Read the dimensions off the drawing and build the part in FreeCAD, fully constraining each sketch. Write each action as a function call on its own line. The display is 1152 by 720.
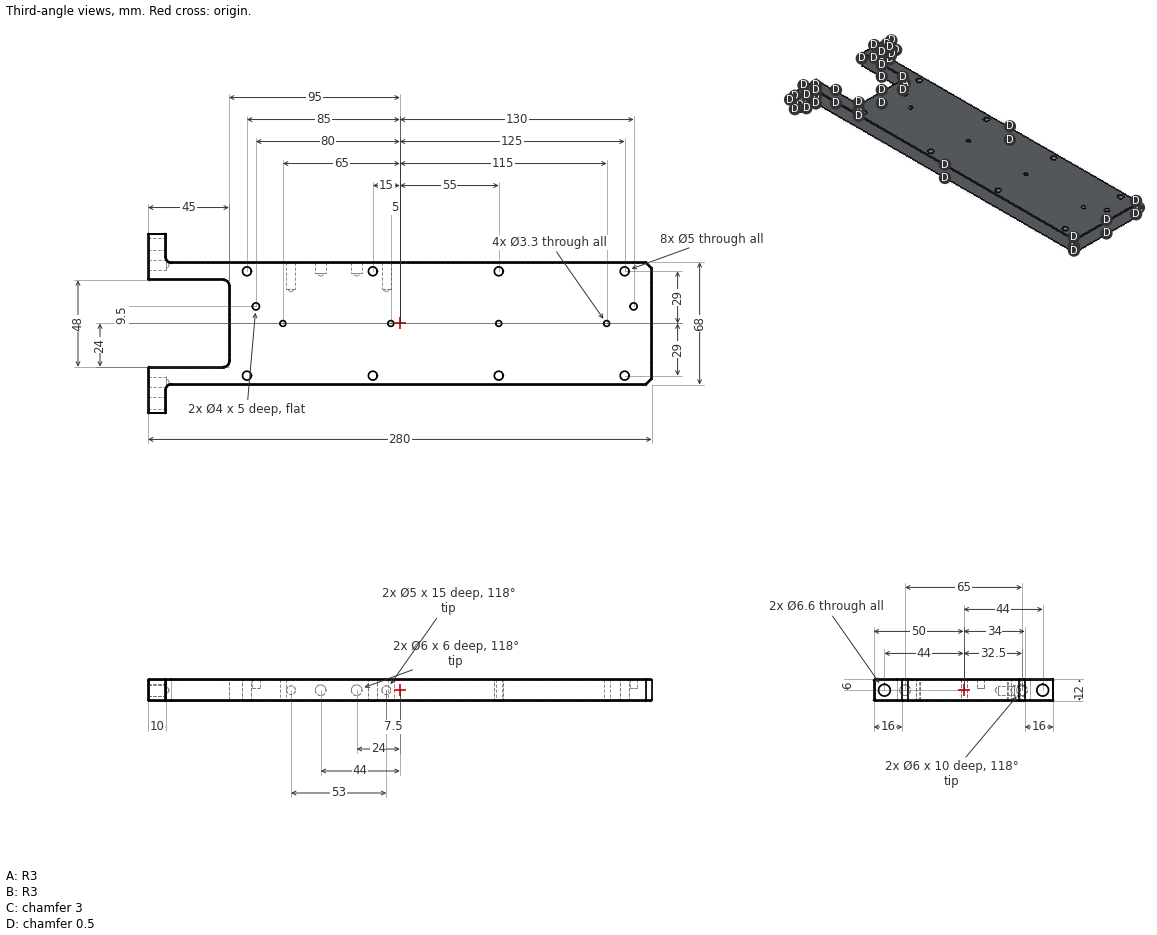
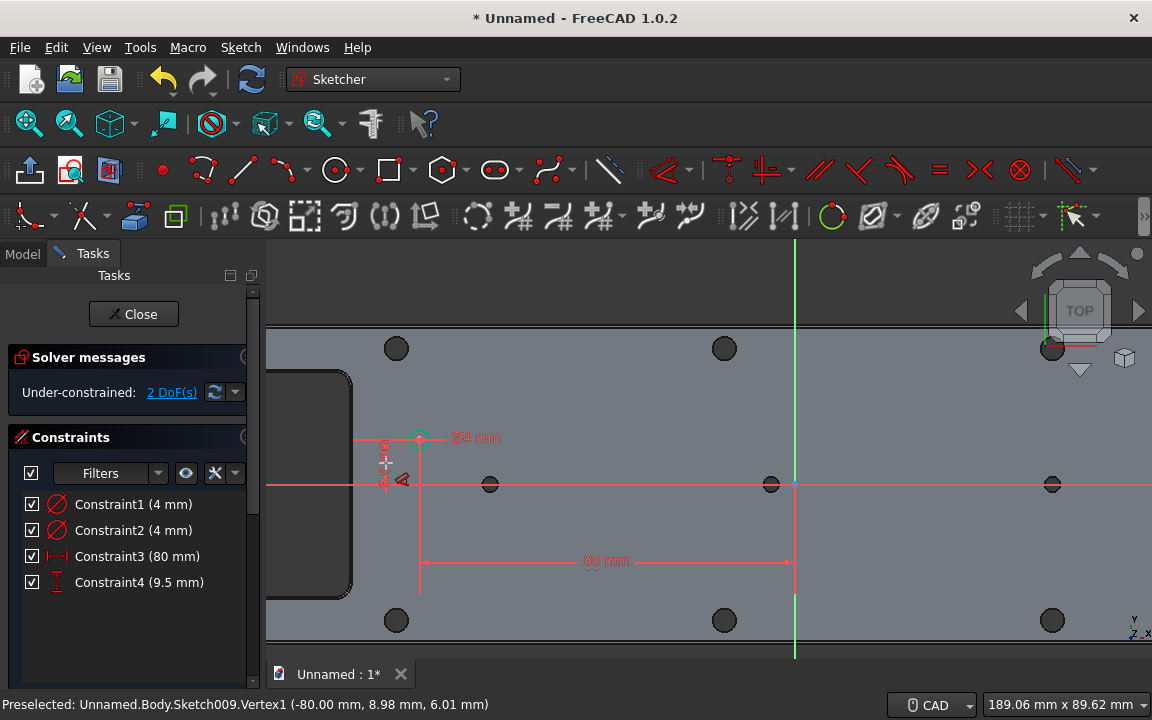
scroll(419, 442, down, 4)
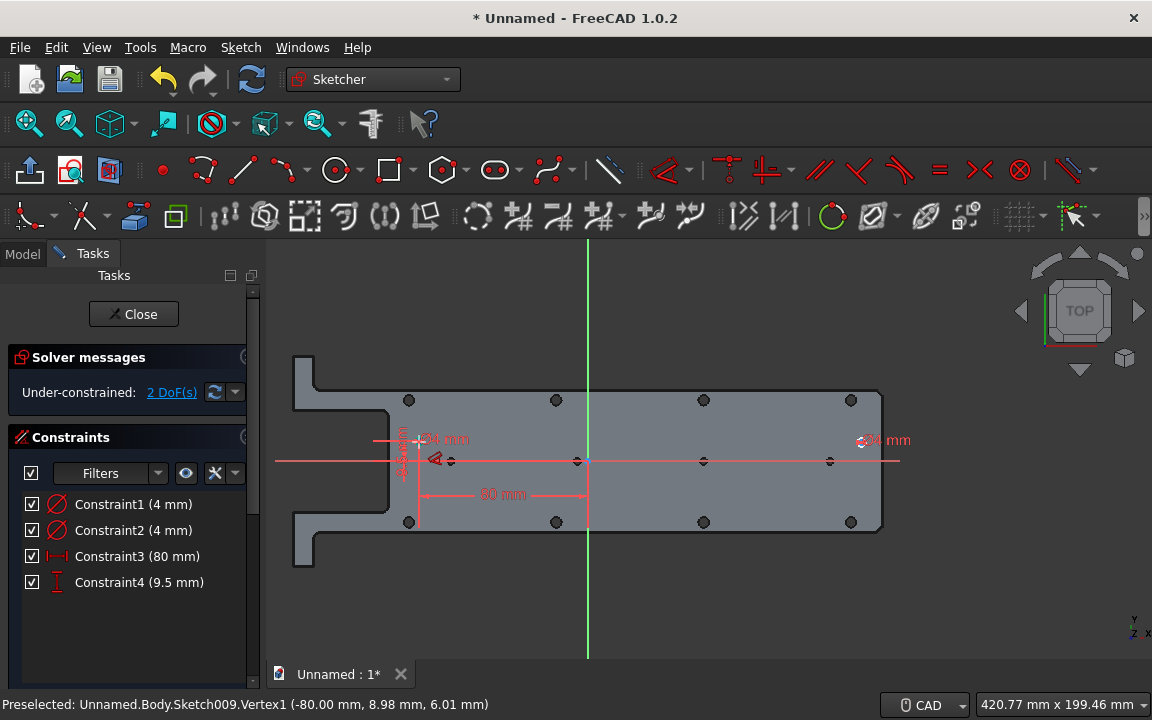
click(861, 442)
click(725, 495)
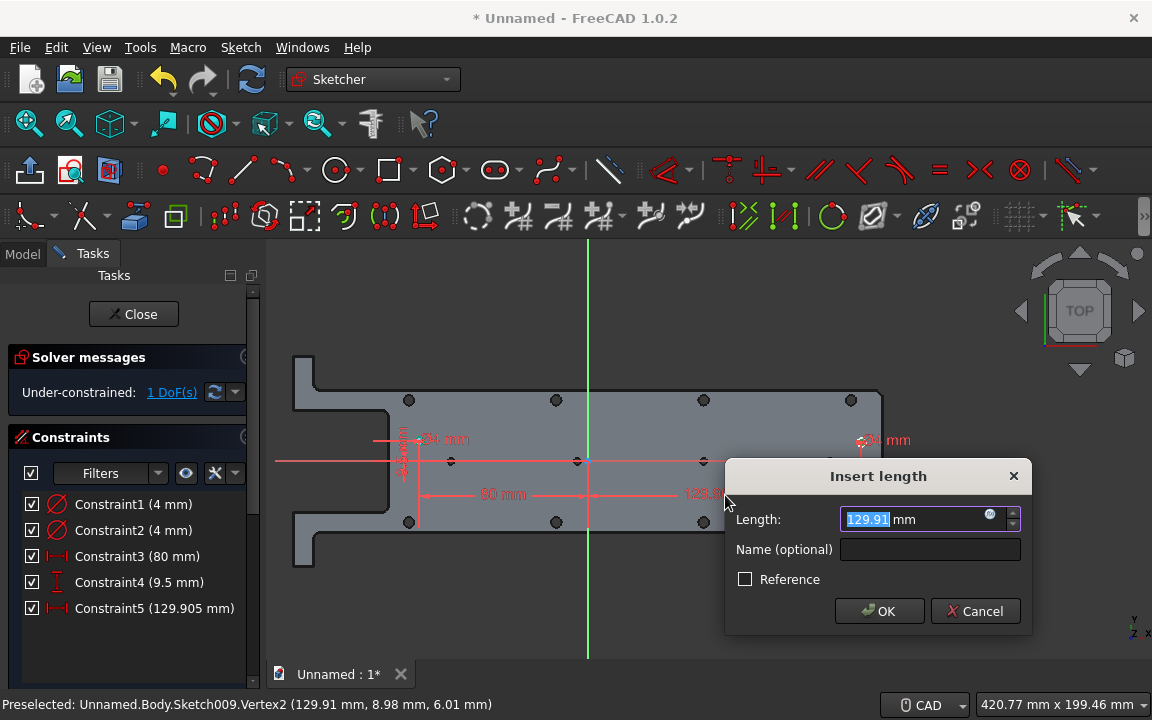
text(130)
key(Return)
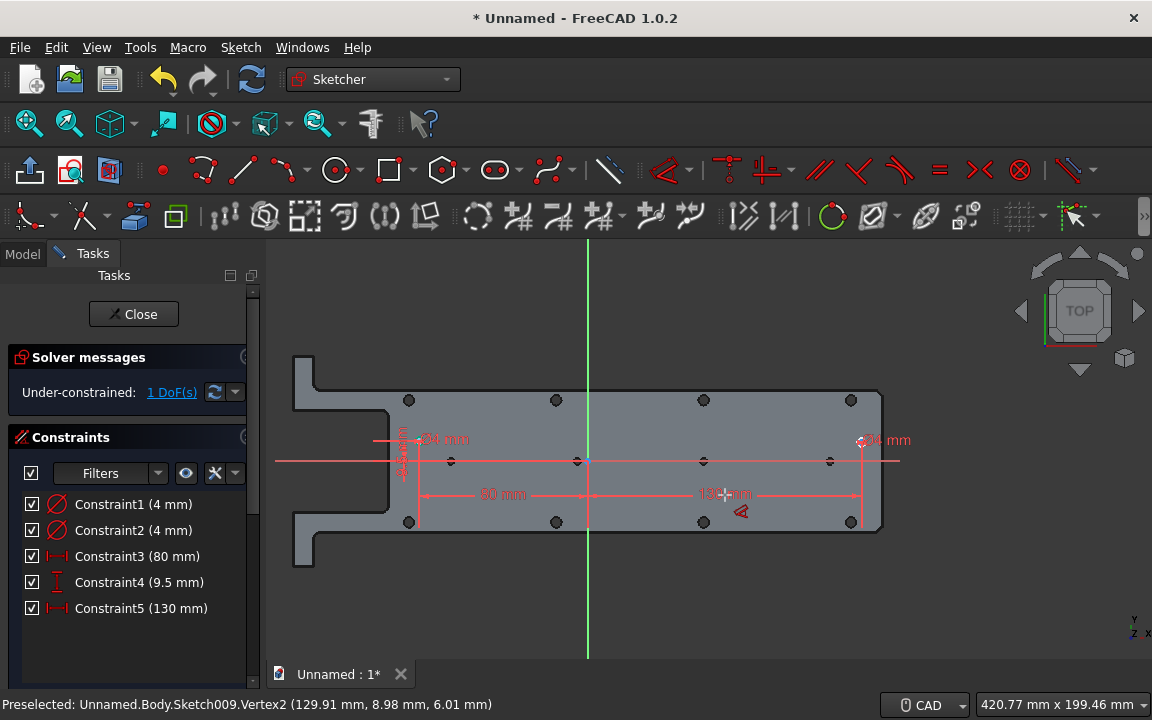
scroll(862, 442, up, 4)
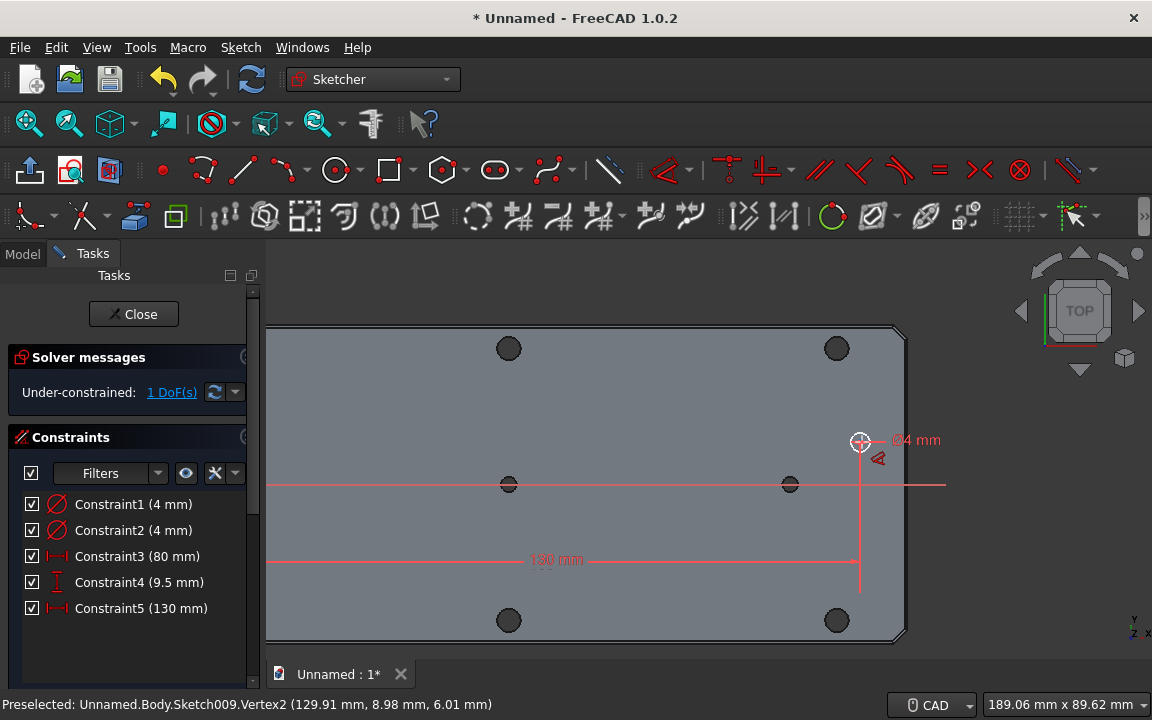
click(860, 442)
click(894, 463)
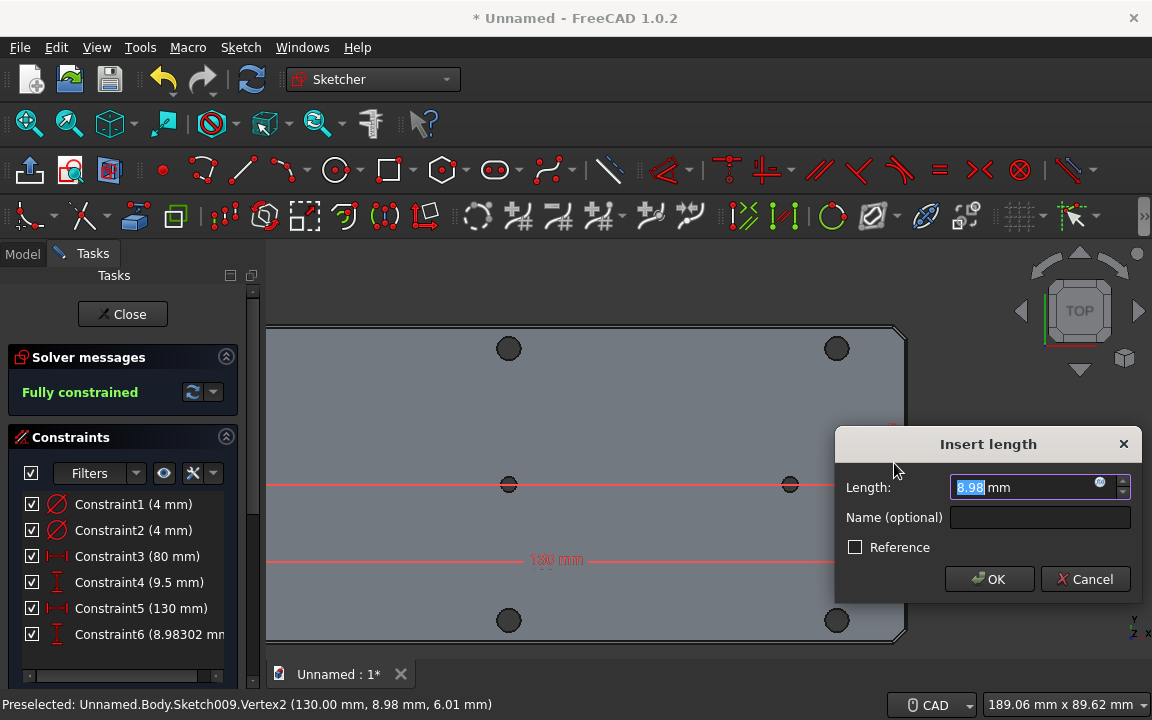
text(9.5)
key(Return)
key(Escape)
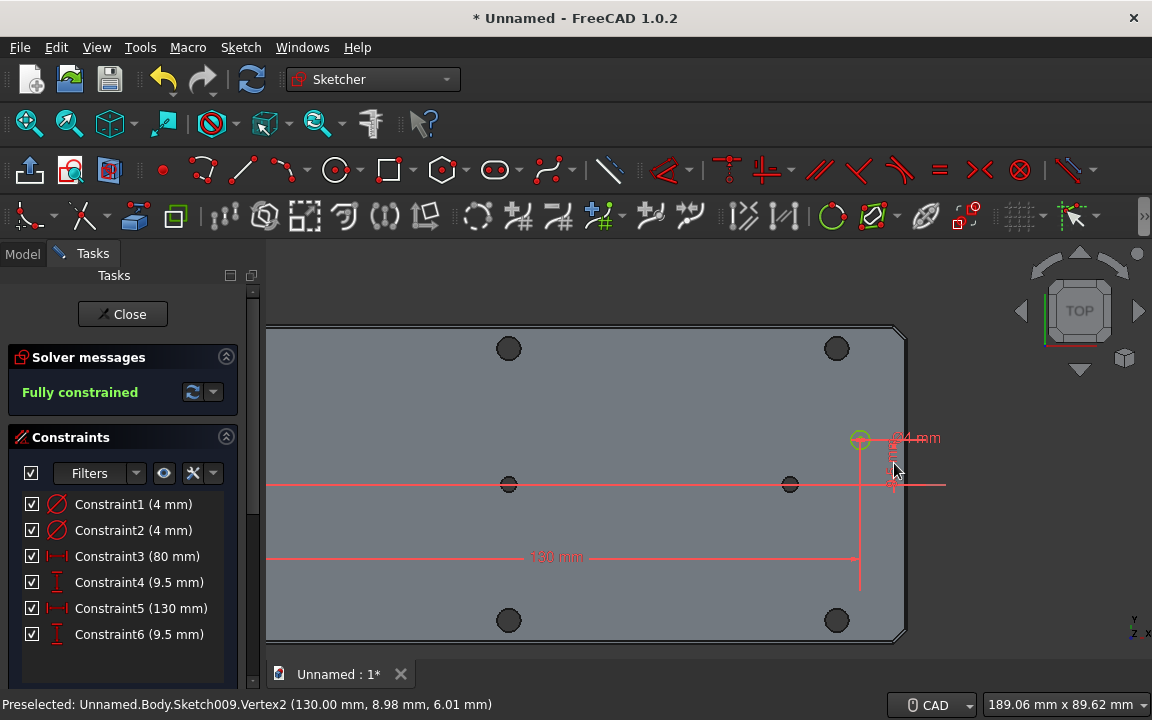
click(123, 314)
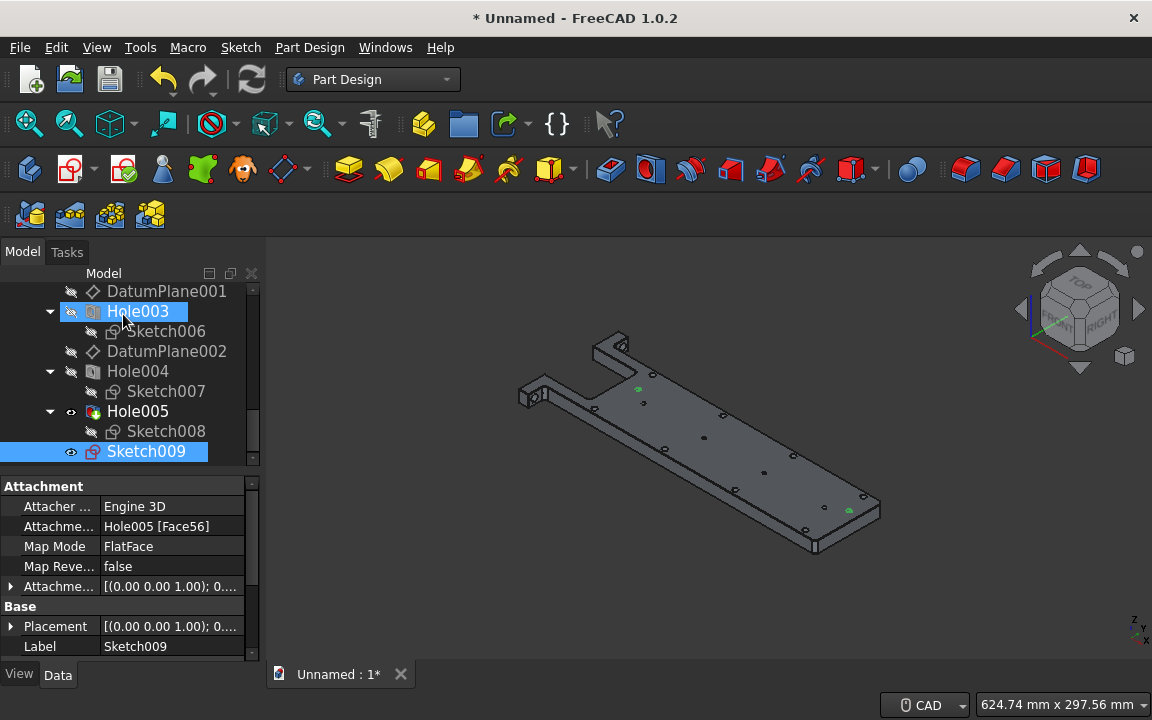
click(652, 170)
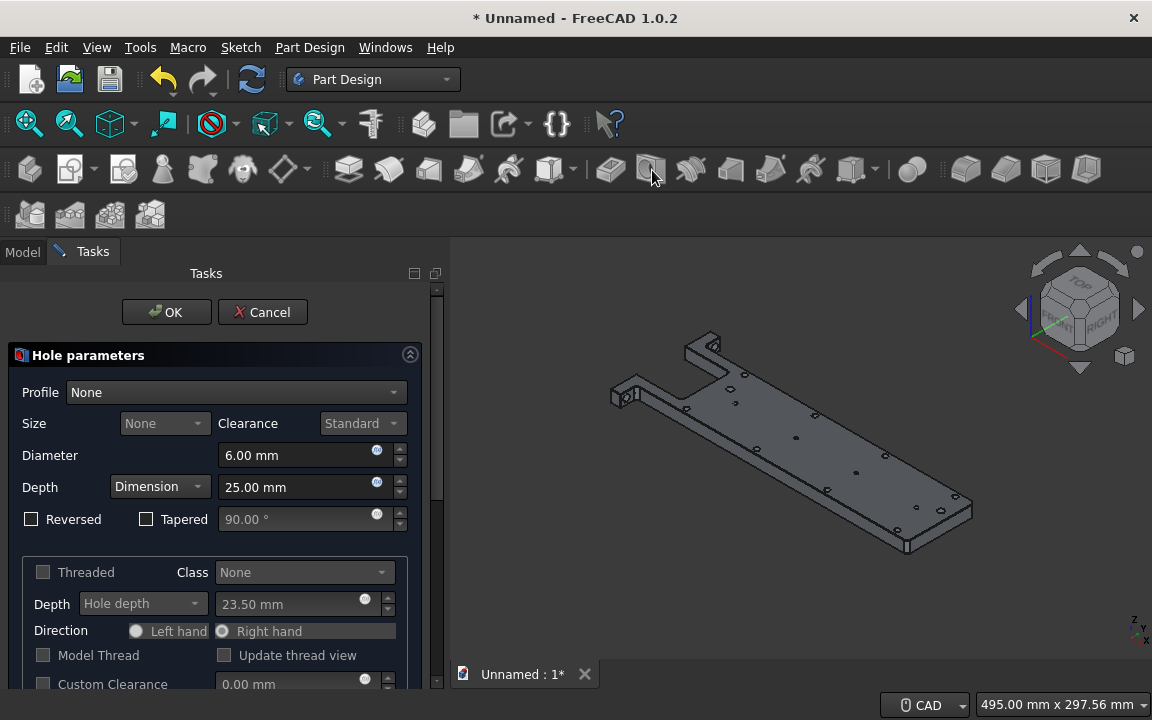
triple_click(305, 455)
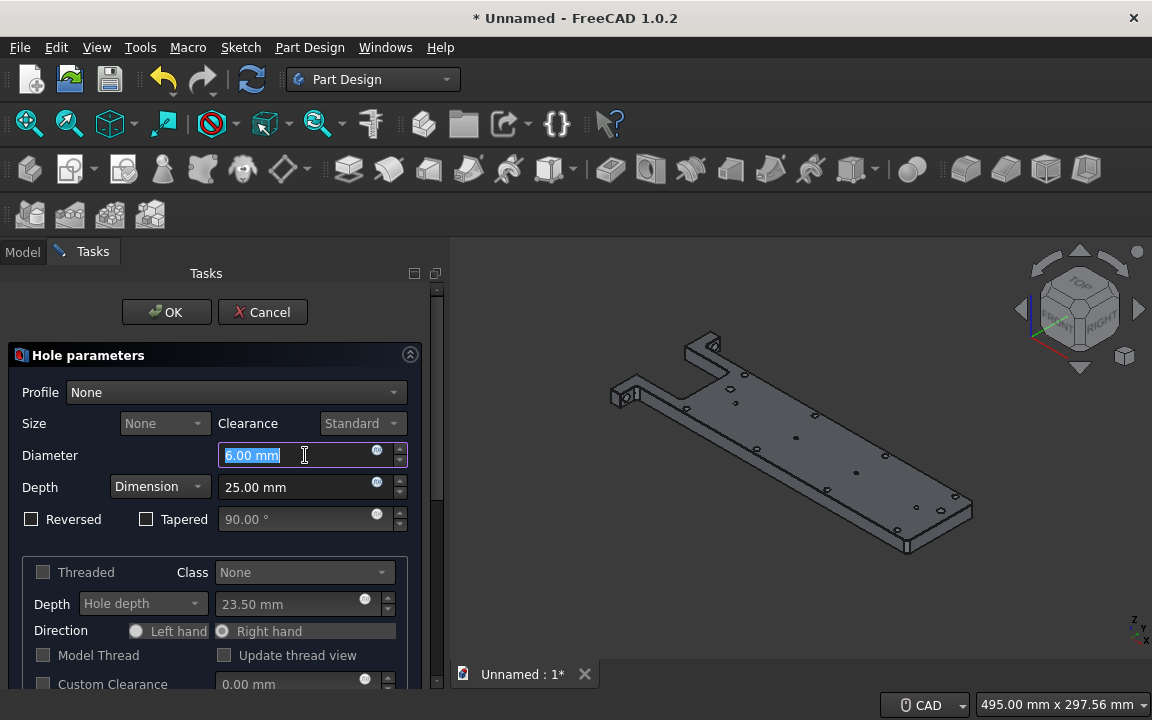
text(4)
key(Tab)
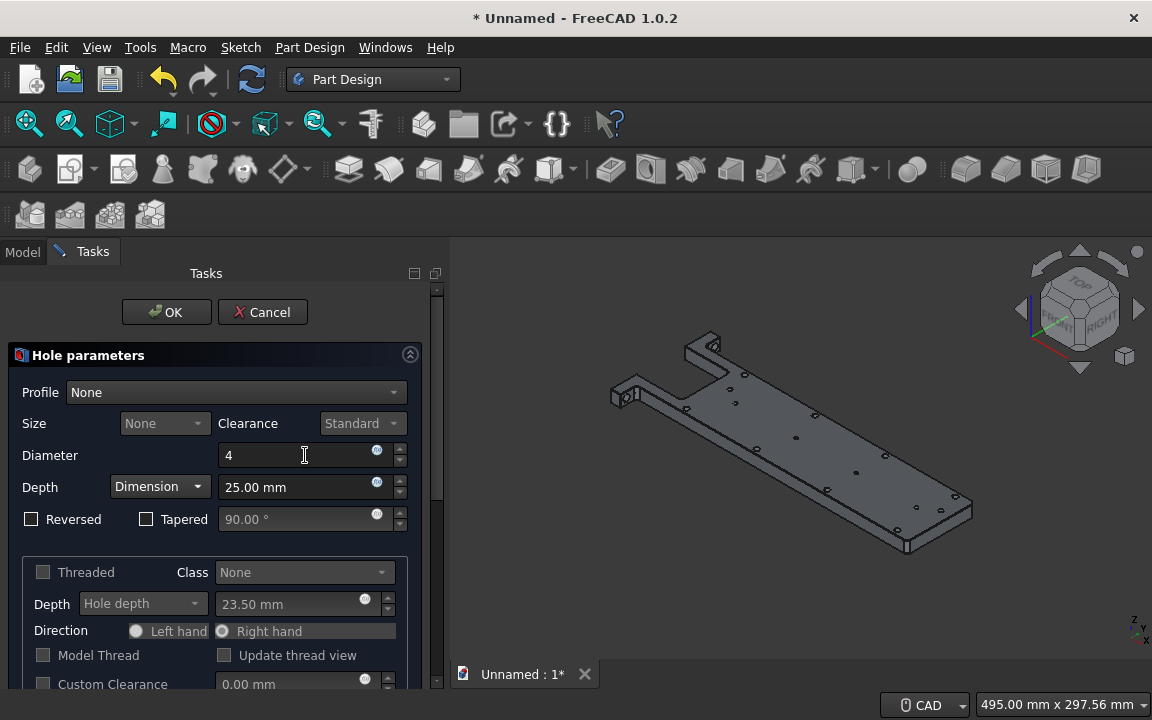
triple_click(305, 487)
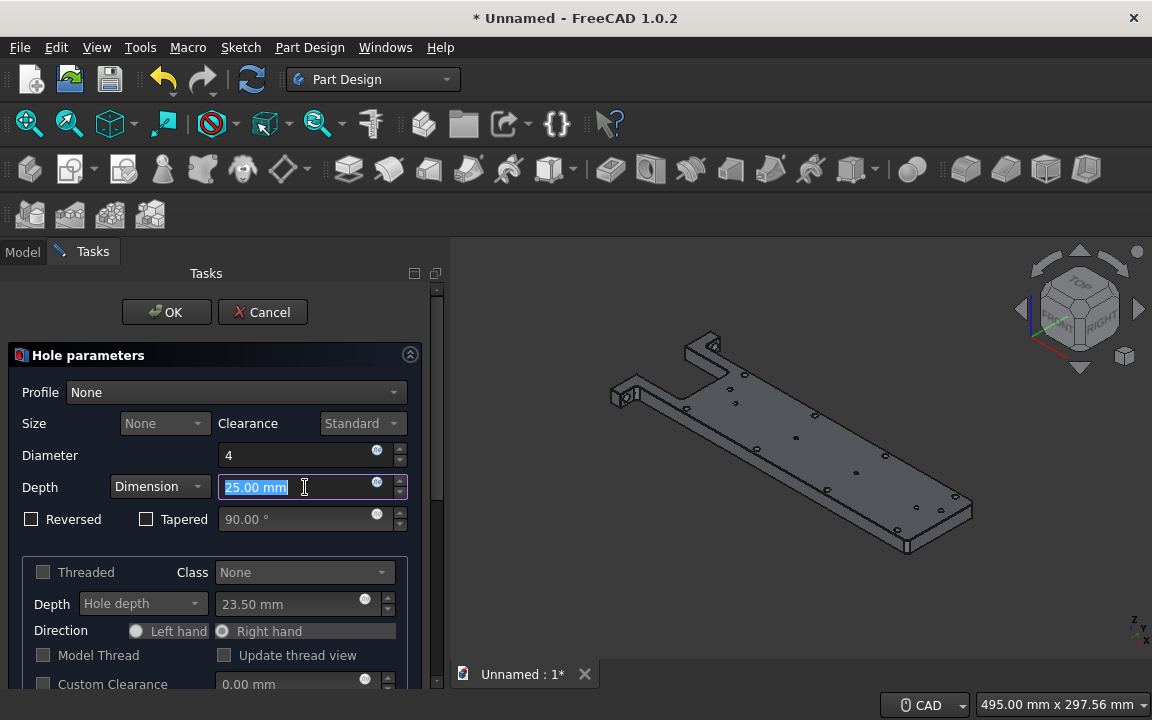
text(5)
key(Tab)